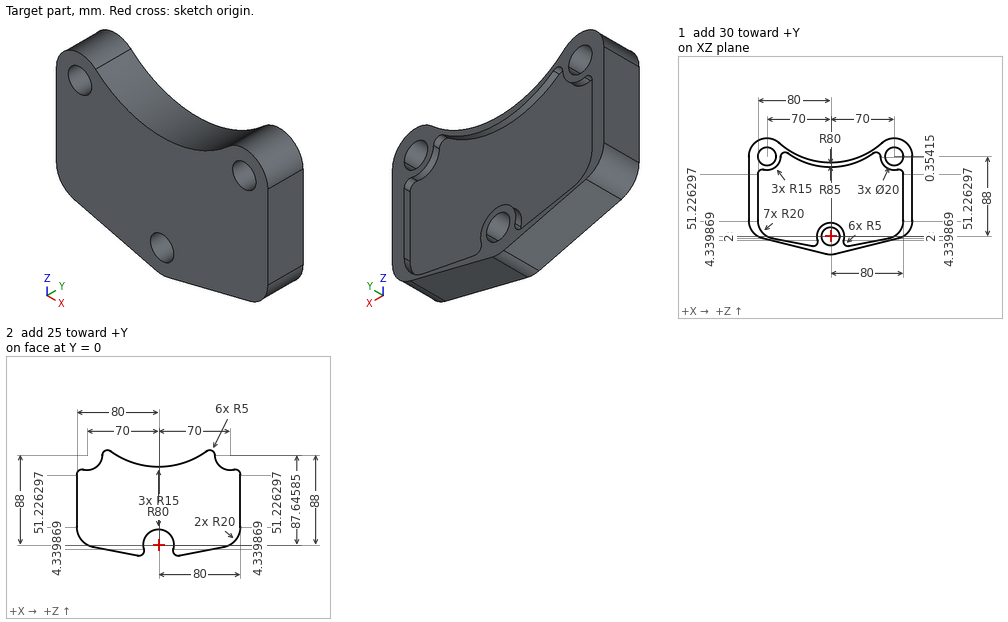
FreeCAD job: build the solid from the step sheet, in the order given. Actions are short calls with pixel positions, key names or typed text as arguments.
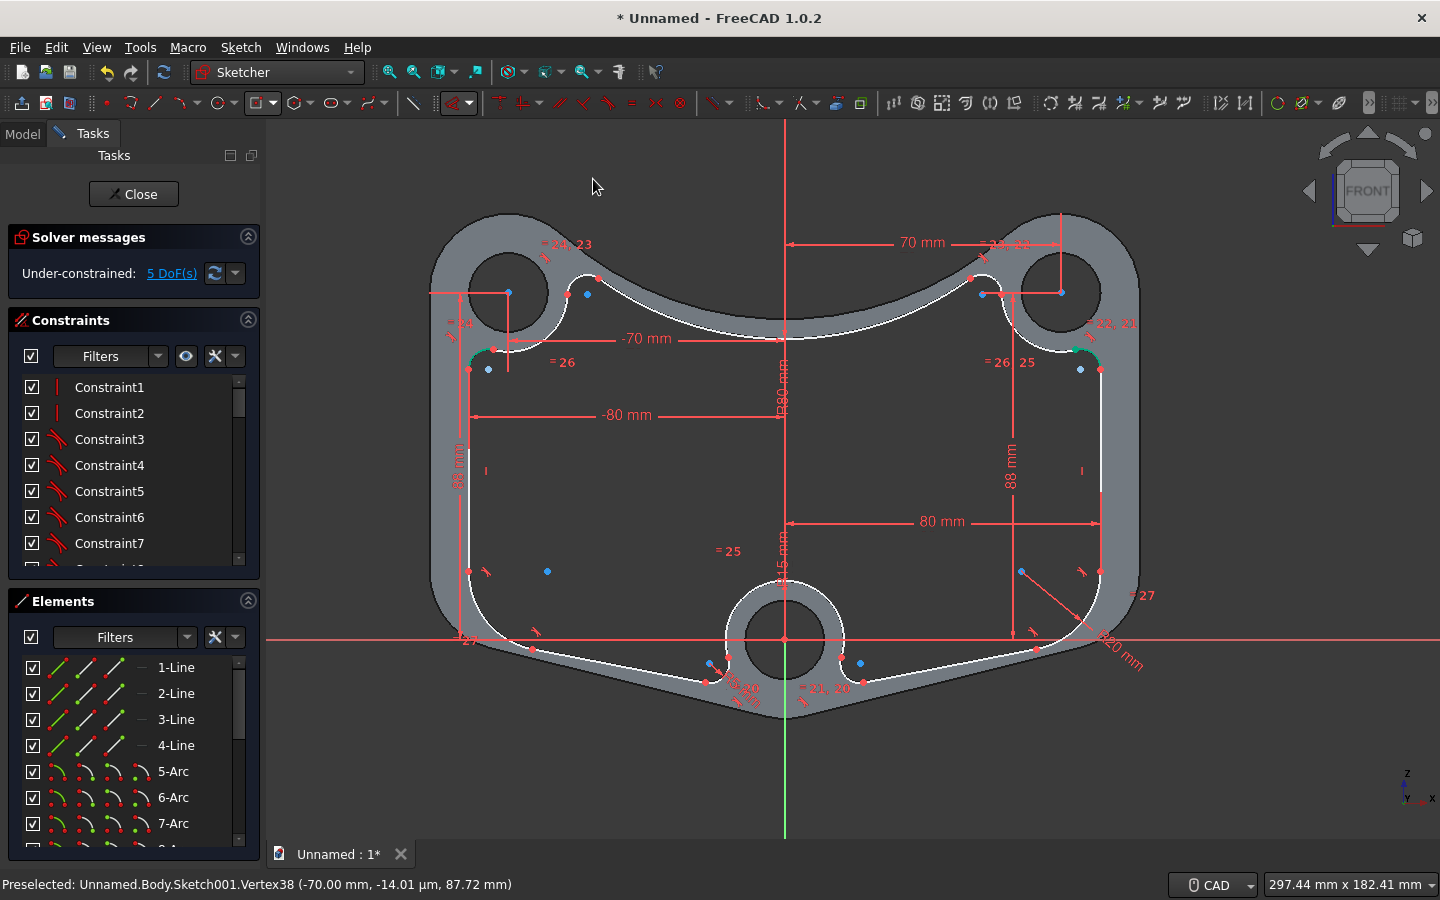
click(1101, 511)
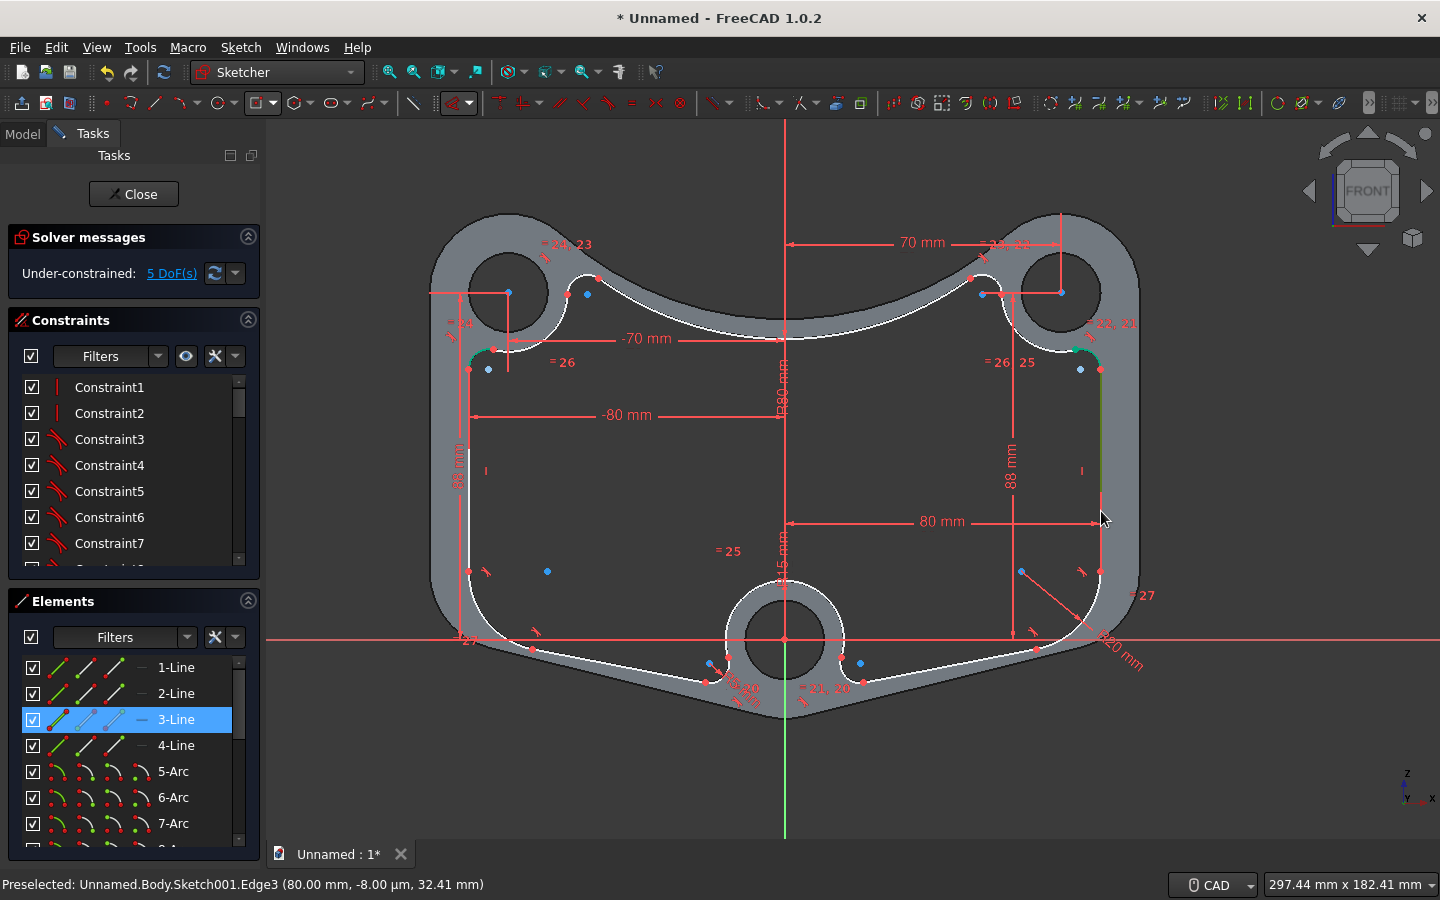
click(472, 104)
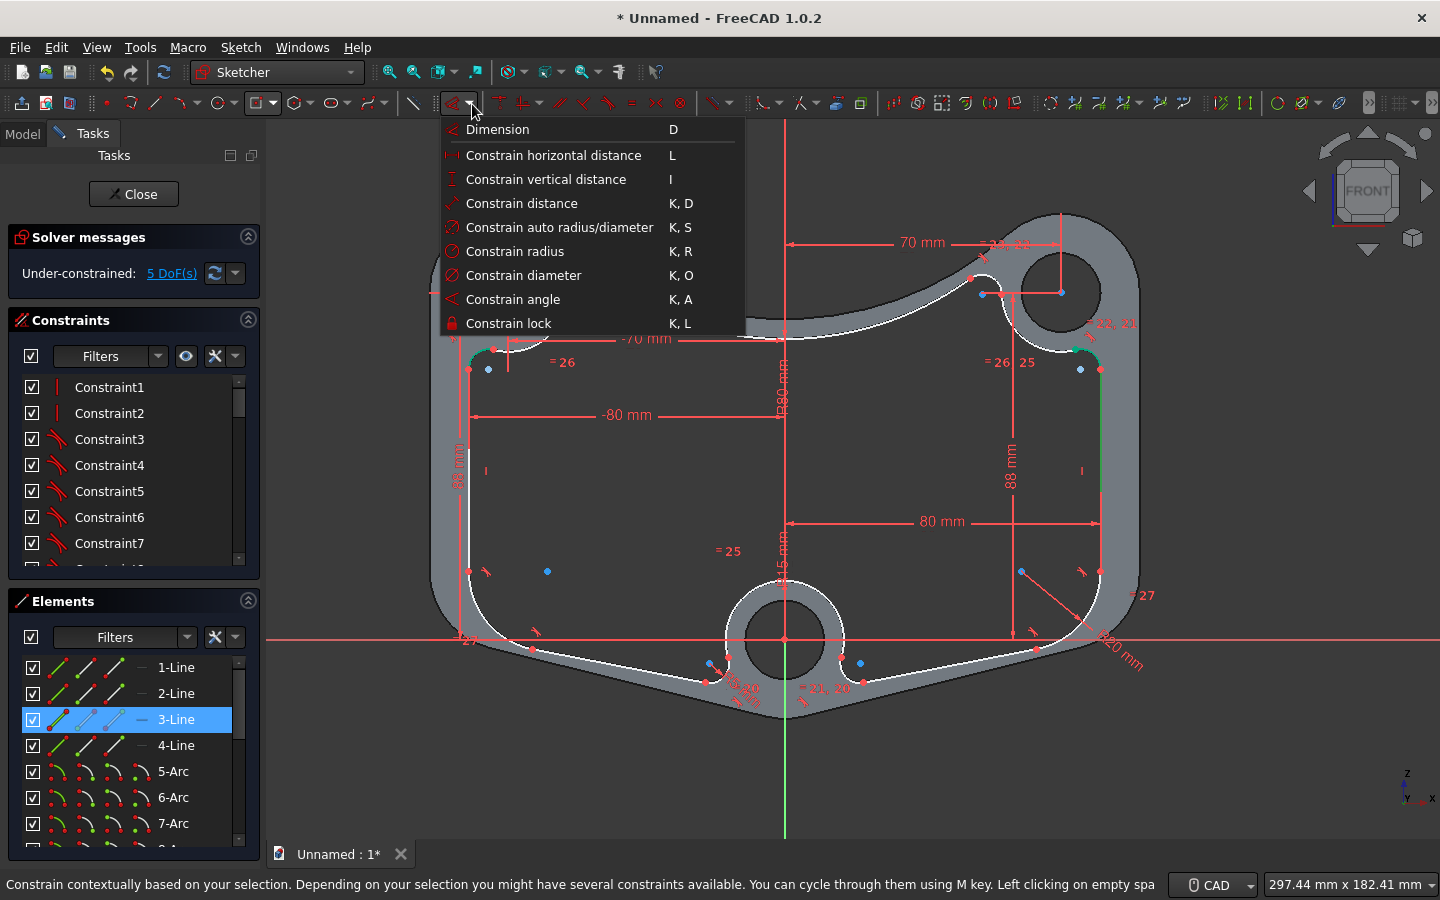
click(593, 179)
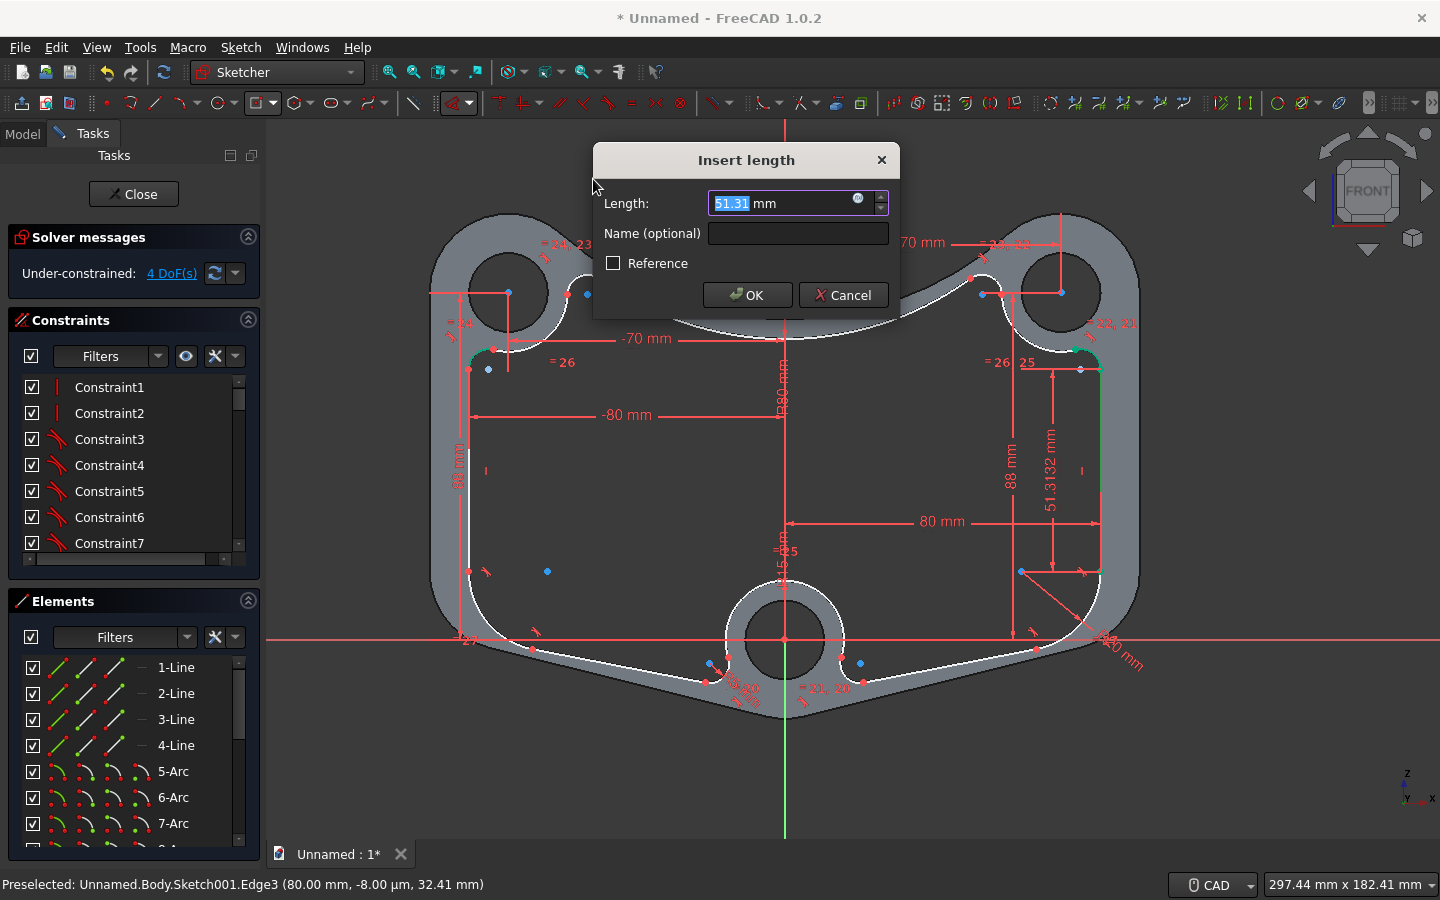
text(51.226297)
key(Return)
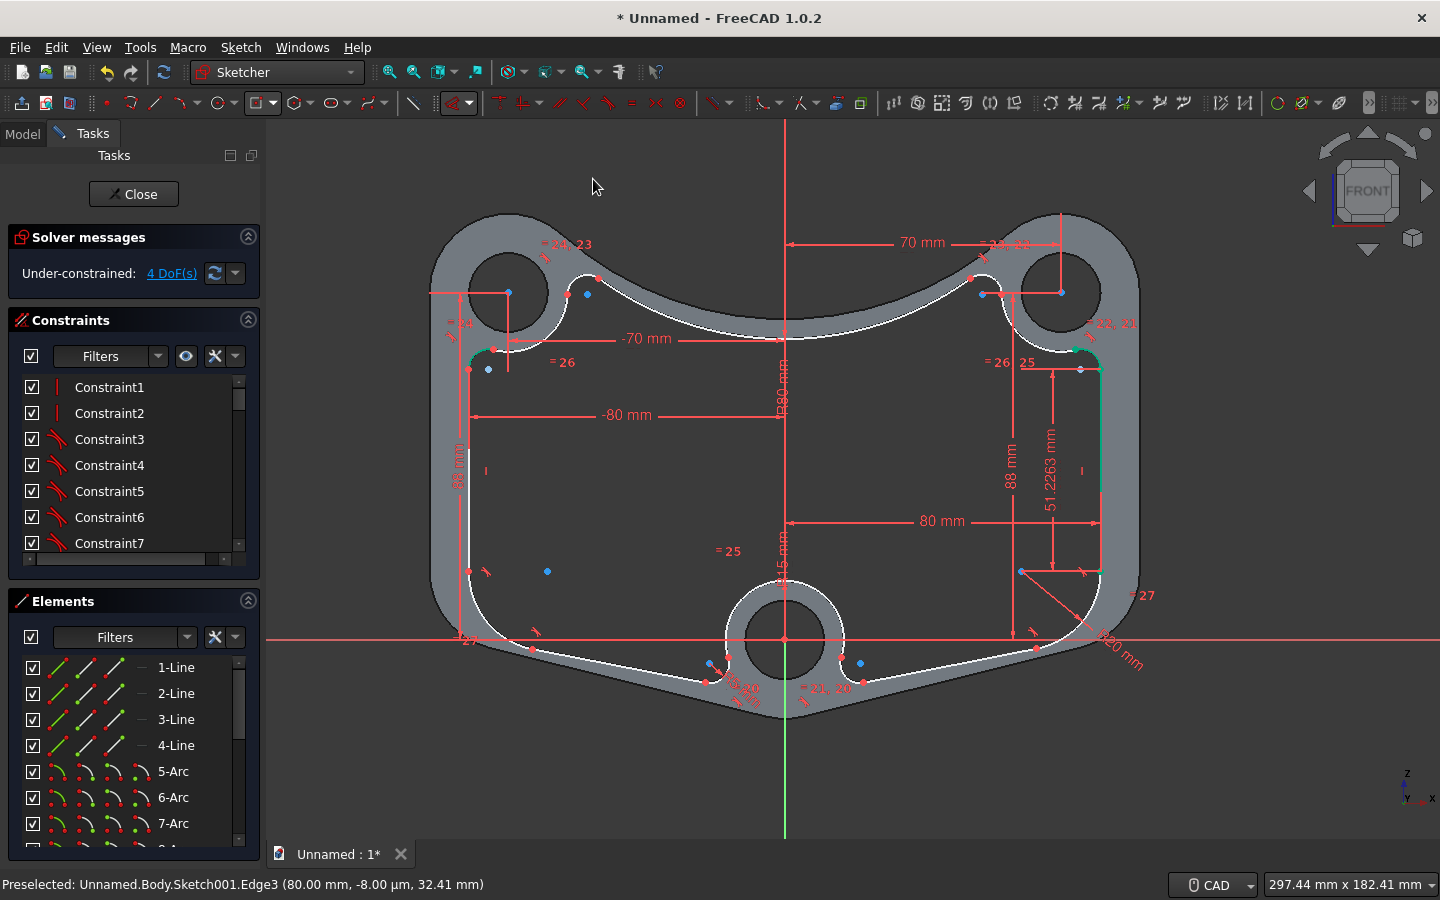
click(469, 430)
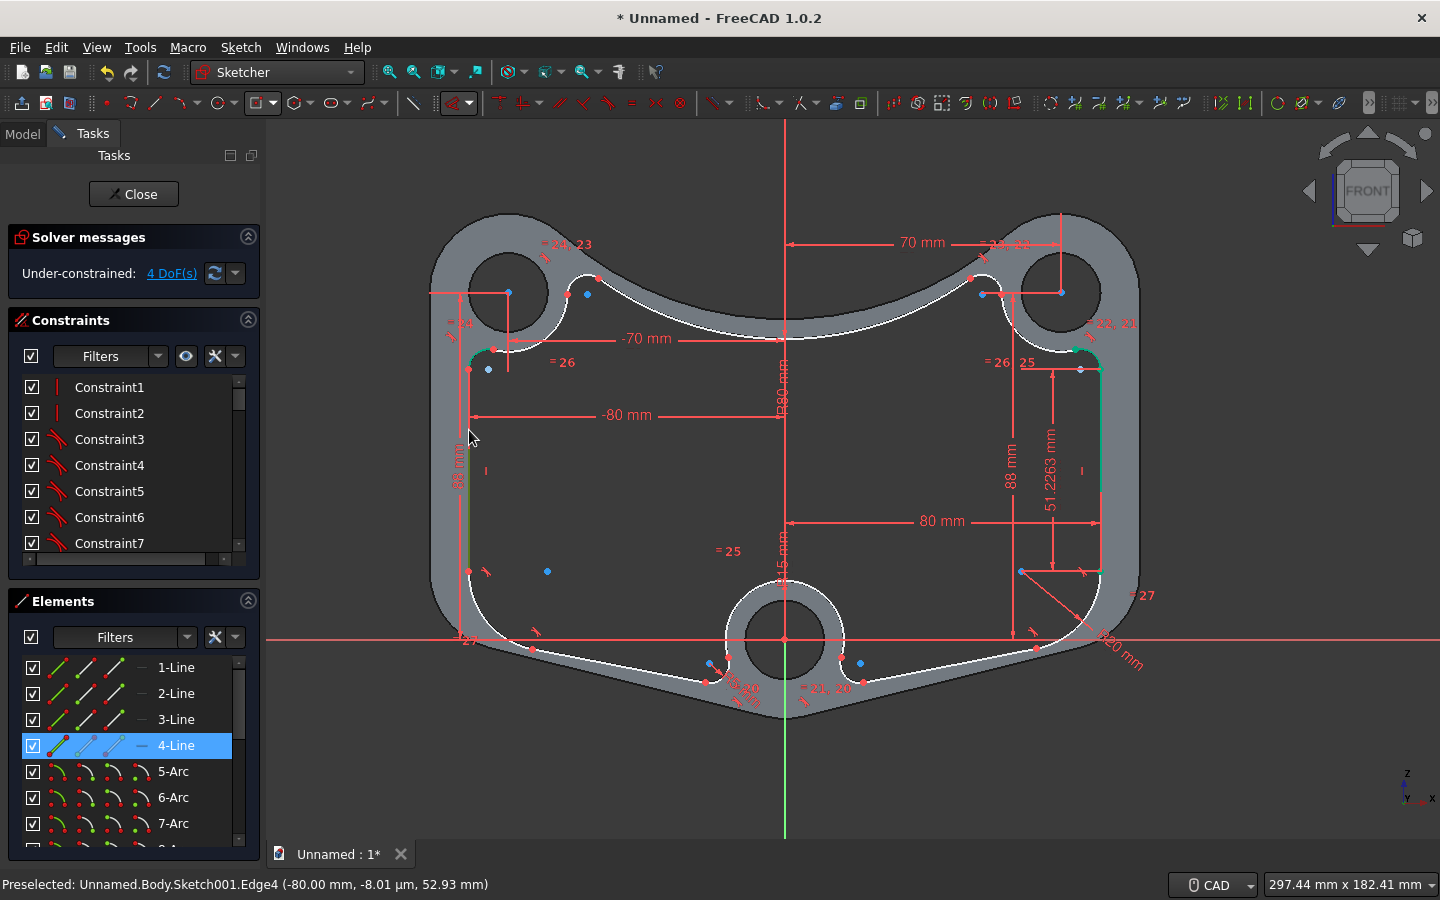
key(i)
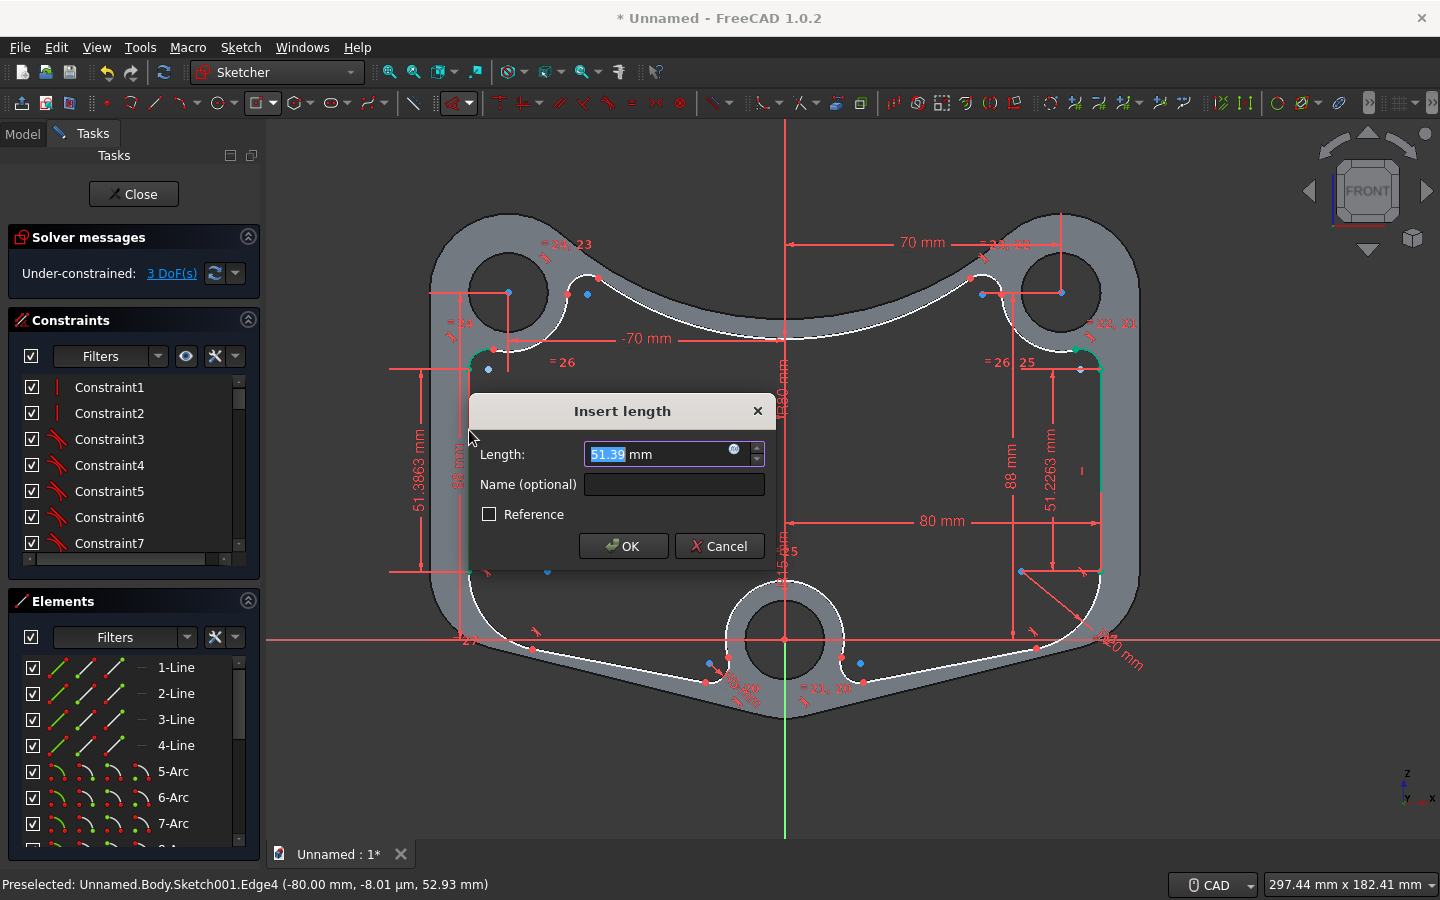
text(51.226297)
key(Return)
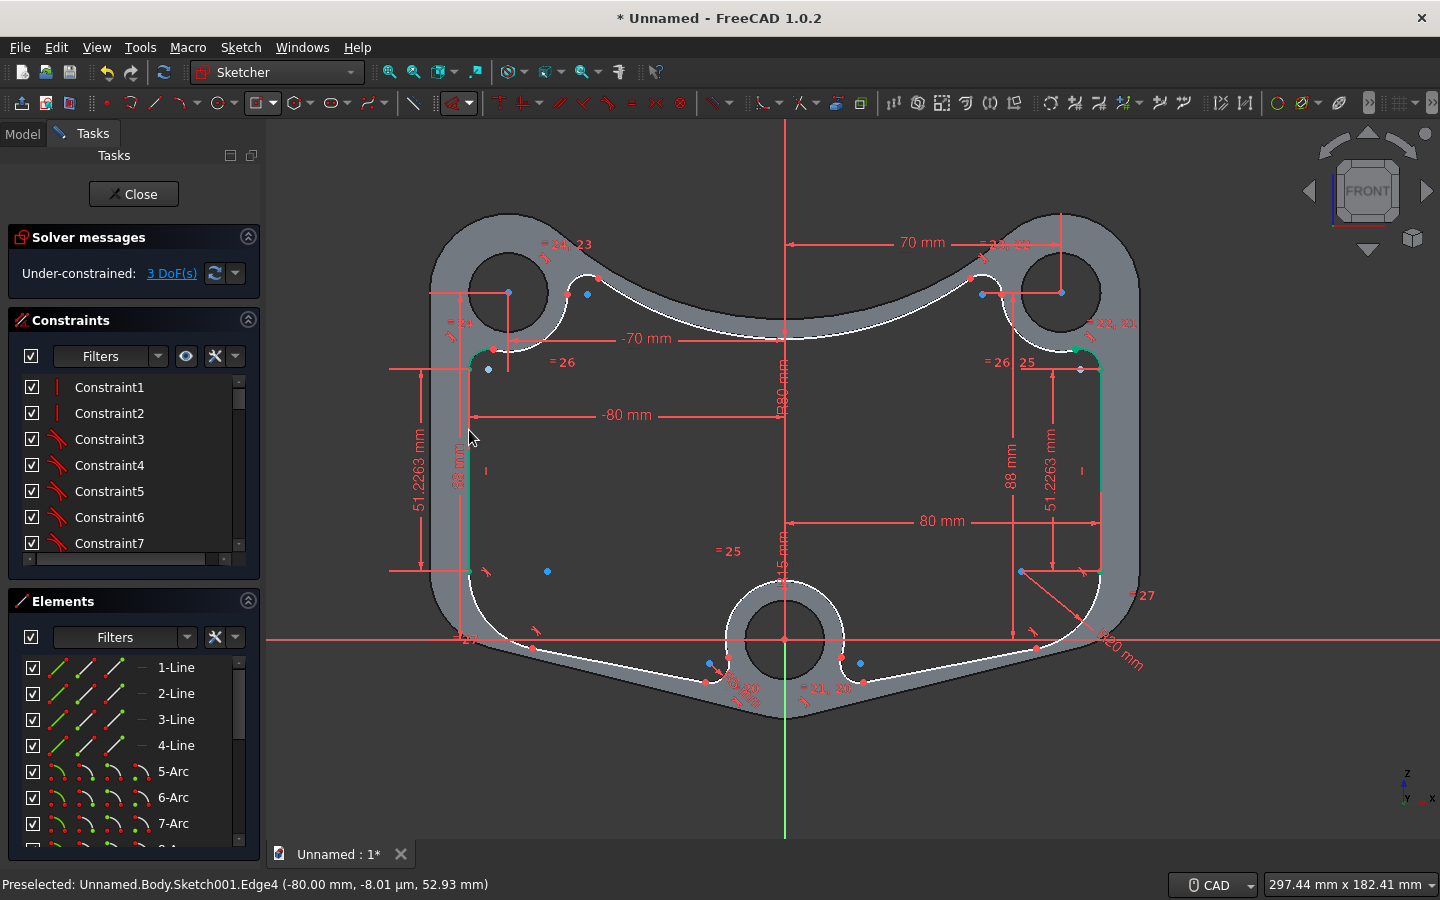
scroll(728, 658, up, 5)